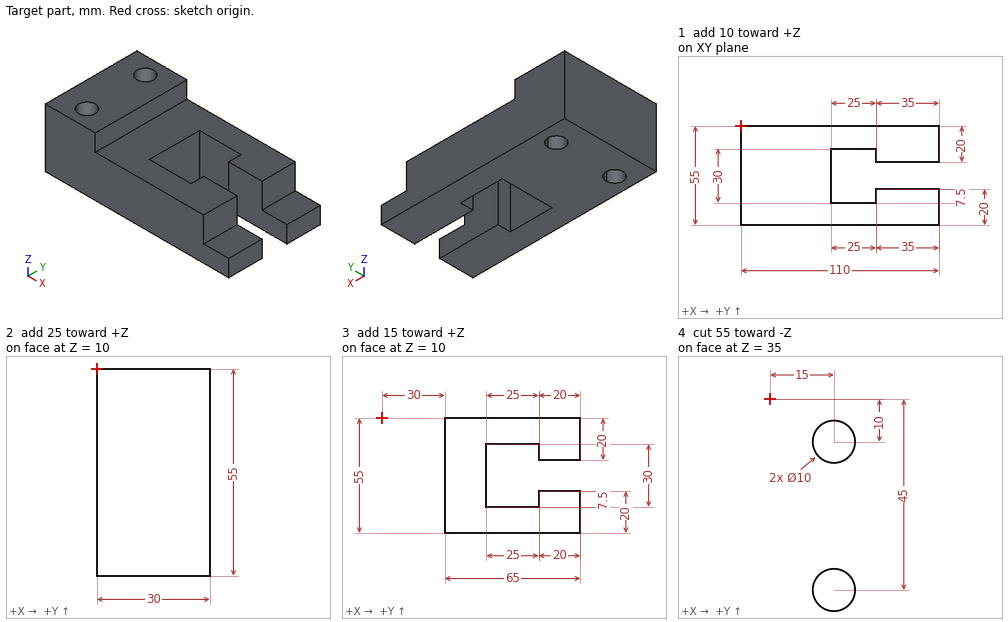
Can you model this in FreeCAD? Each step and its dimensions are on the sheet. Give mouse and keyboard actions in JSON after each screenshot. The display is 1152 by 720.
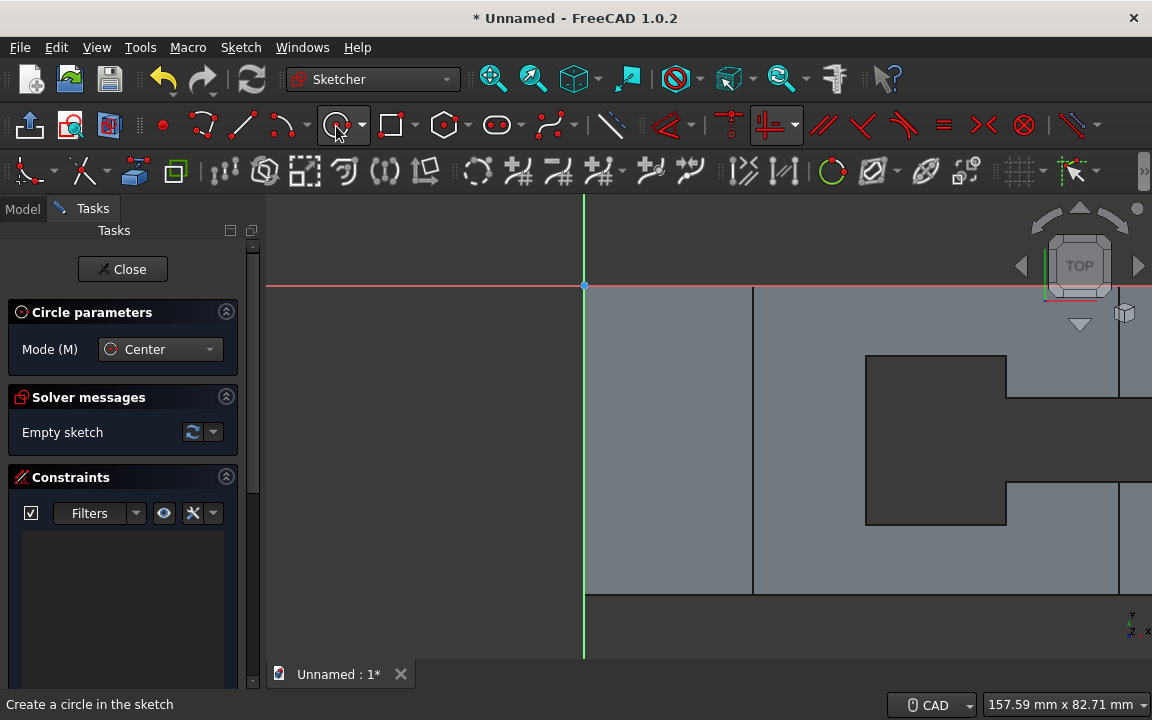
{"action": "left_click", "coordinate": [669, 342]}
{"action": "mouse_move", "coordinate": [689, 322]}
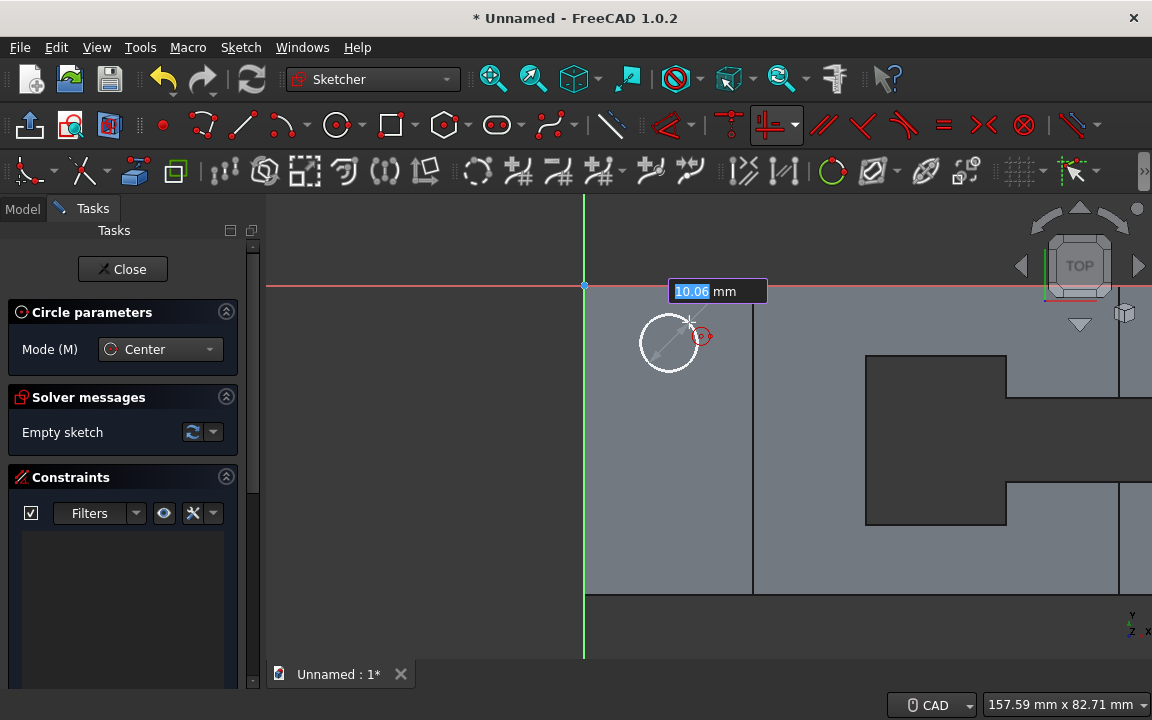
{"action": "type", "text": "10"}
{"action": "key", "text": "Return"}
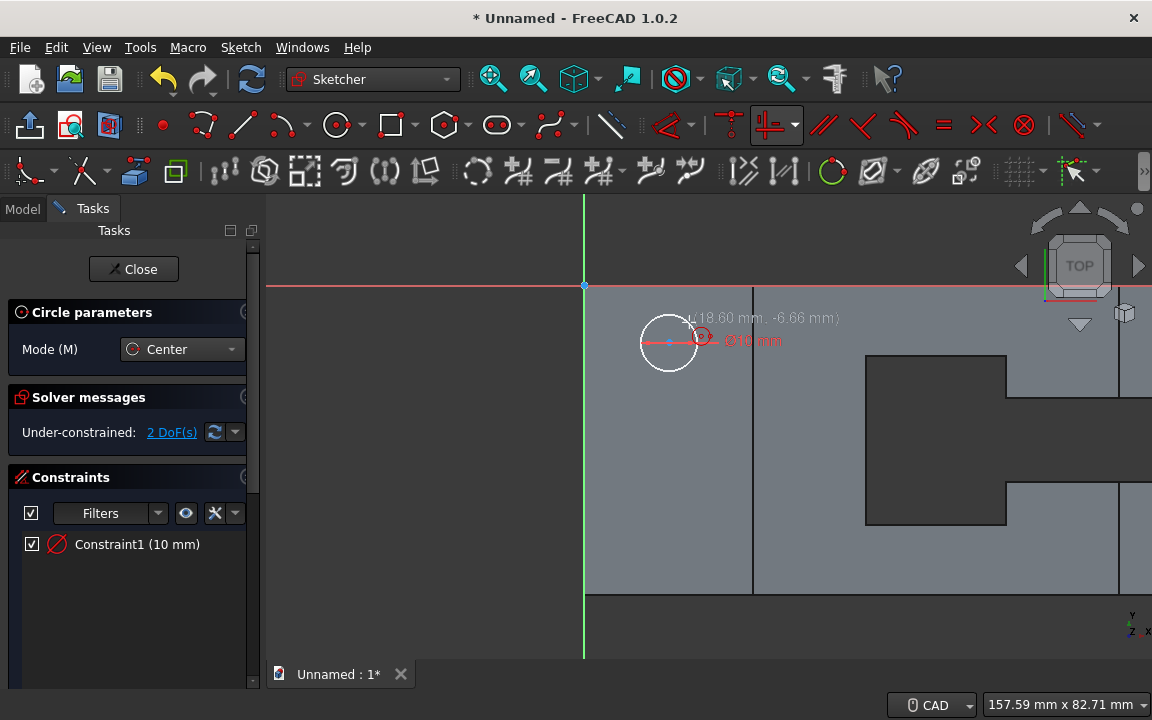
{"action": "left_click", "coordinate": [669, 539]}
{"action": "mouse_move", "coordinate": [689, 519]}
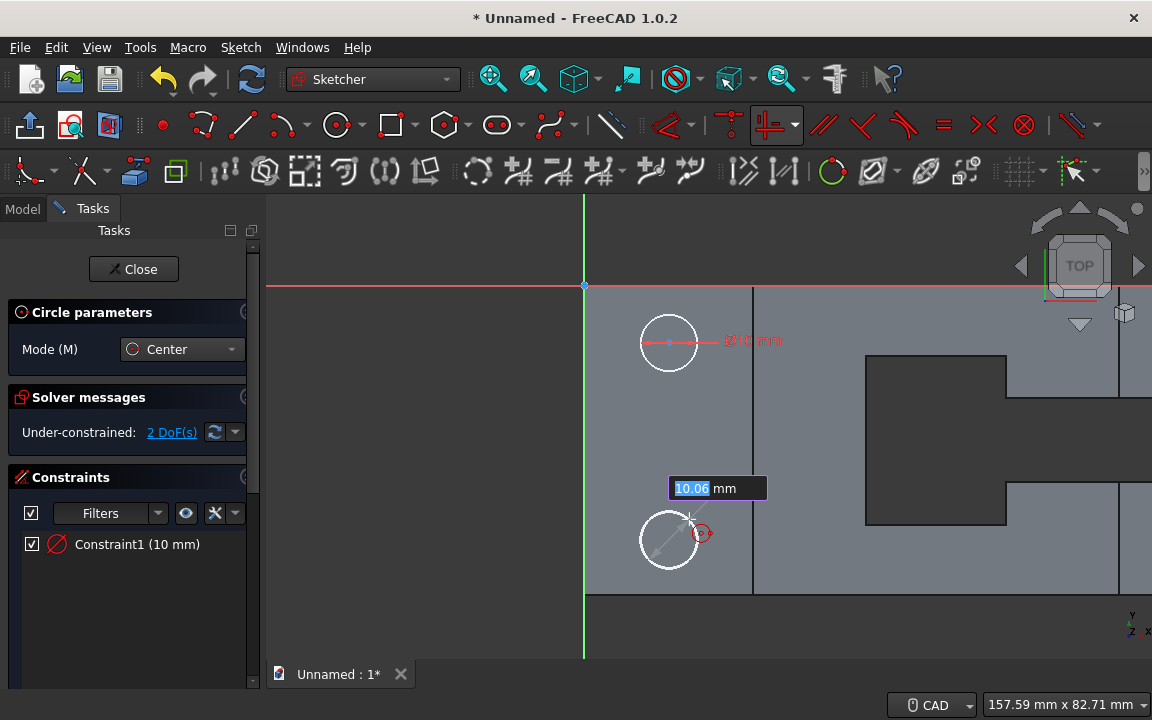
{"action": "type", "text": "10"}
{"action": "key", "text": "Return"}
{"action": "key", "text": "Escape"}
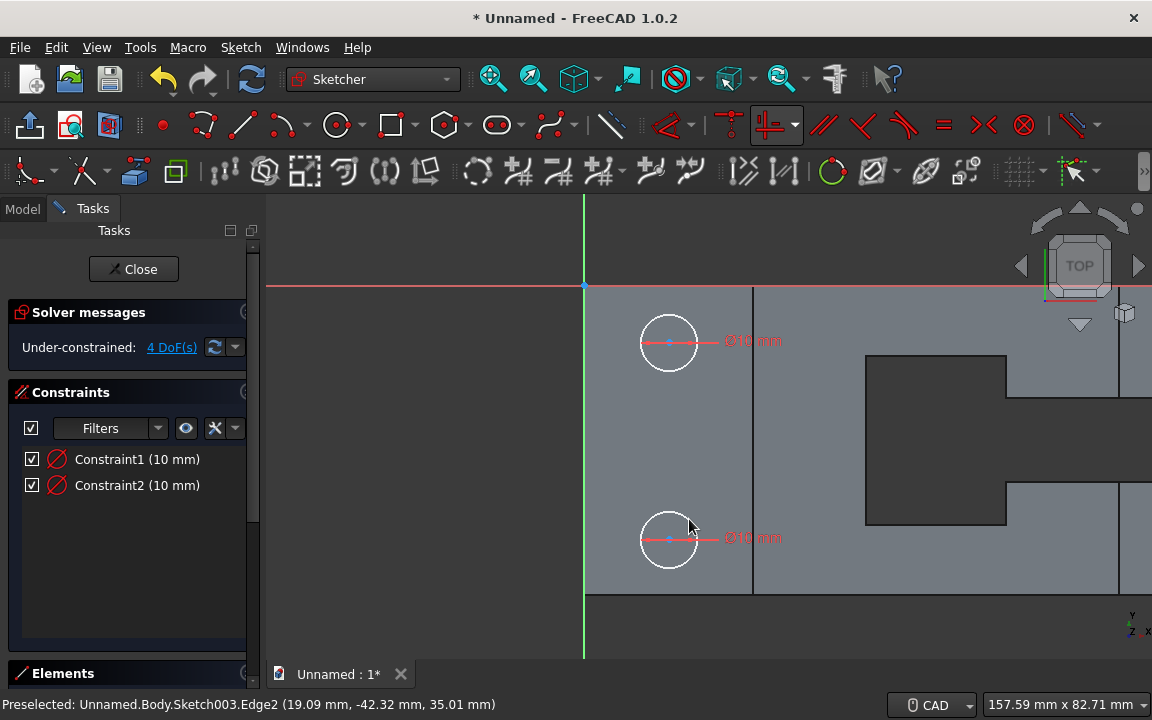
{"action": "left_click", "coordinate": [669, 343]}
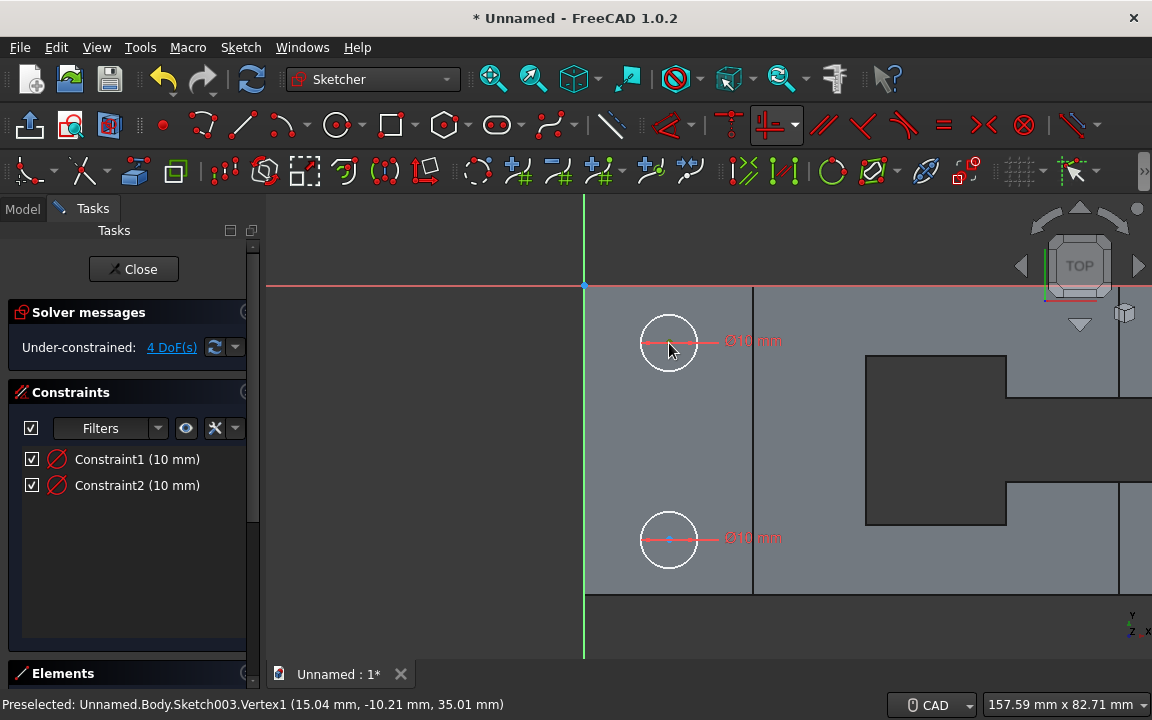
{"action": "left_click", "coordinate": [669, 540]}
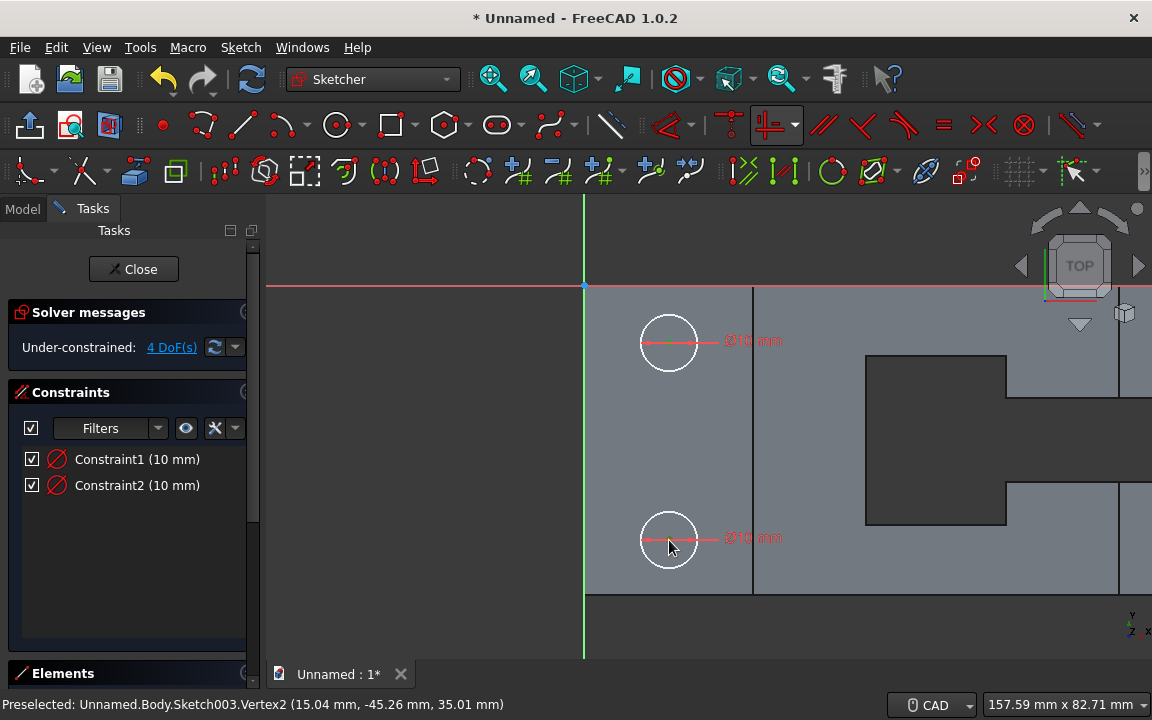
{"action": "left_click", "coordinate": [798, 126]}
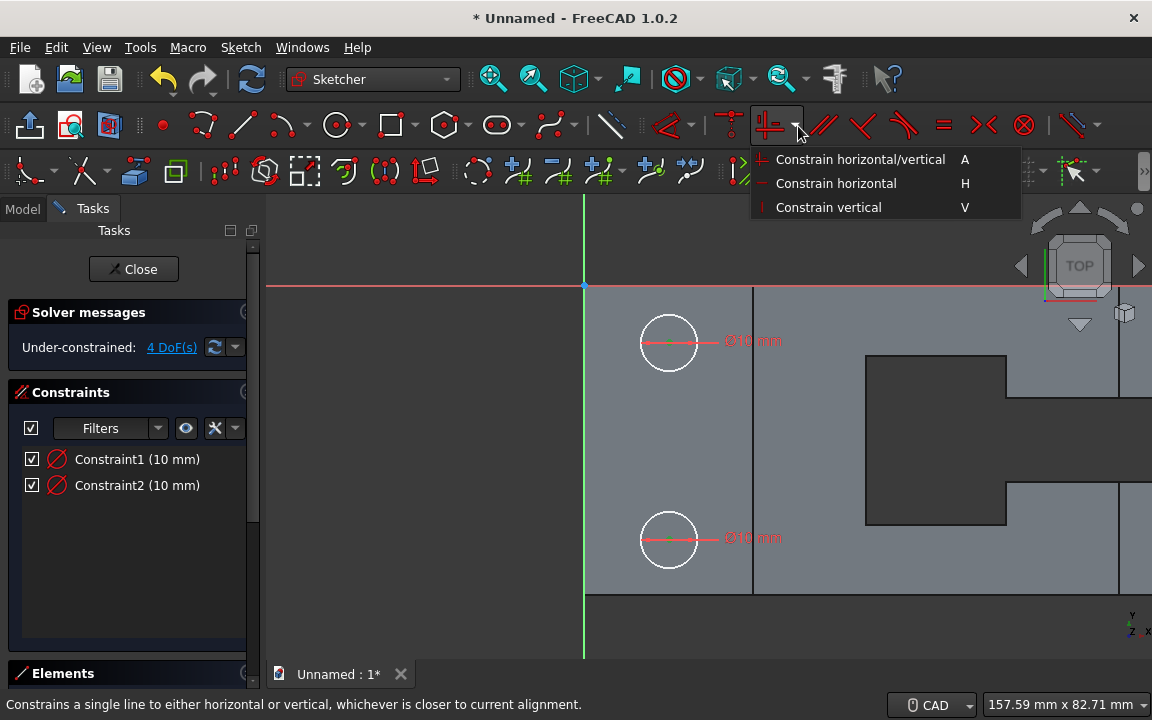
{"action": "left_click", "coordinate": [886, 207]}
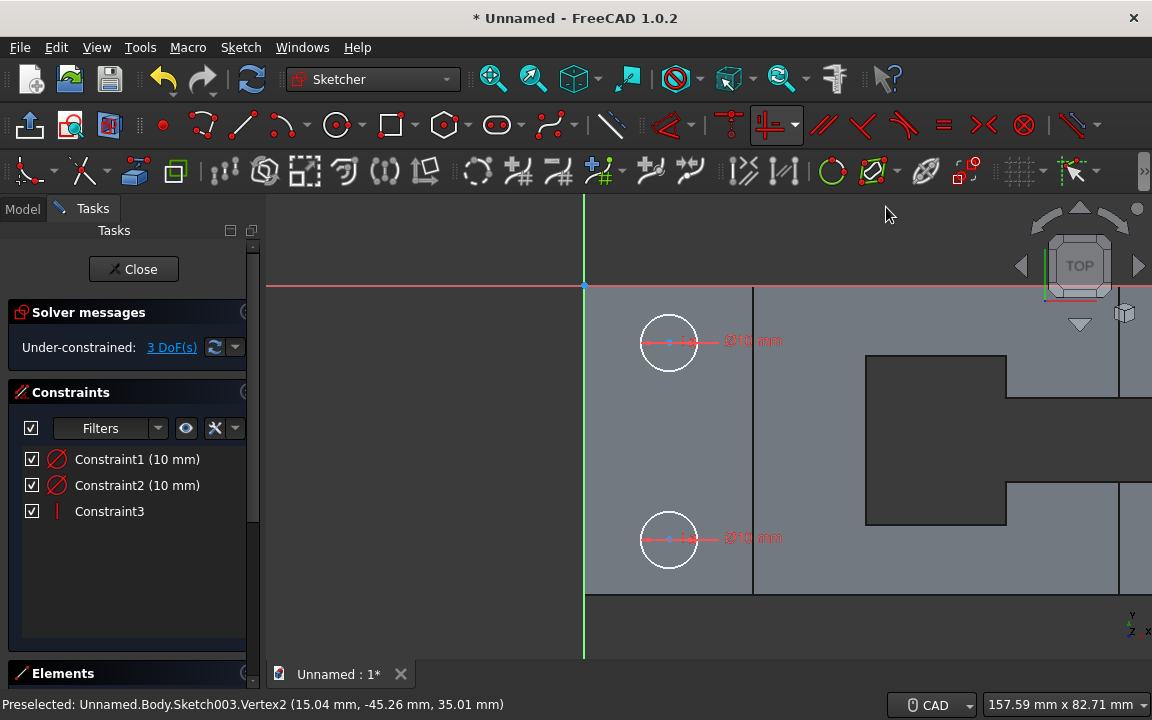
{"action": "left_click", "coordinate": [666, 126]}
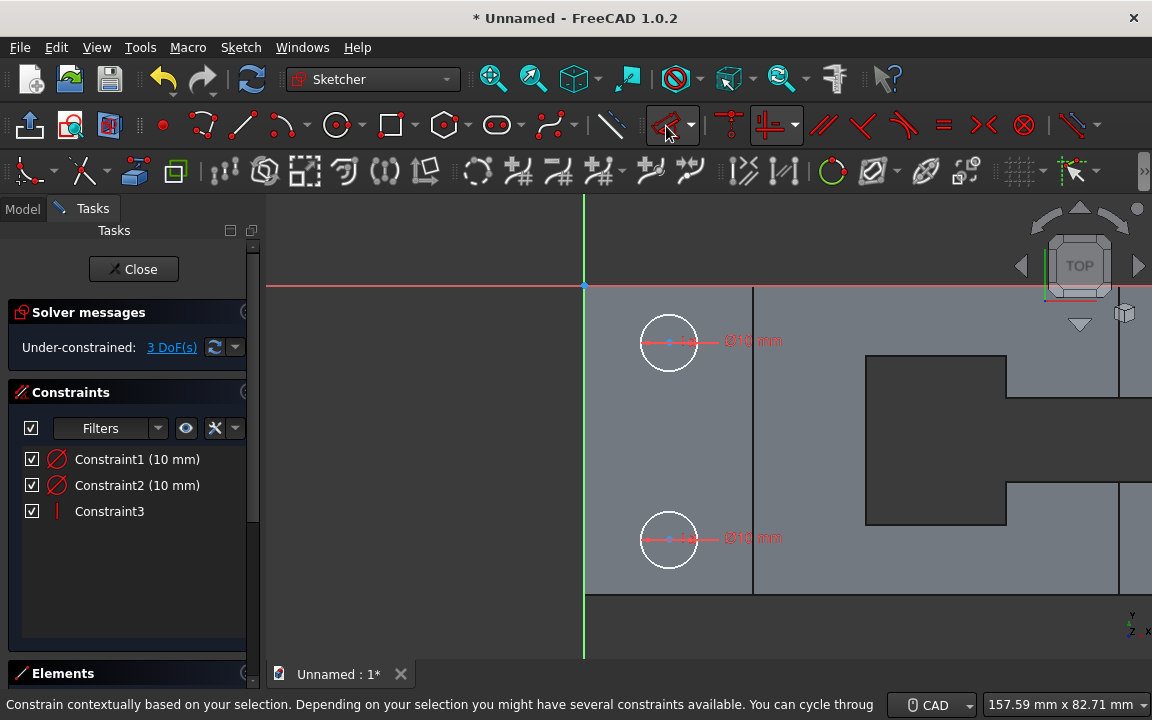
{"action": "left_click", "coordinate": [669, 343]}
{"action": "left_click", "coordinate": [627, 252]}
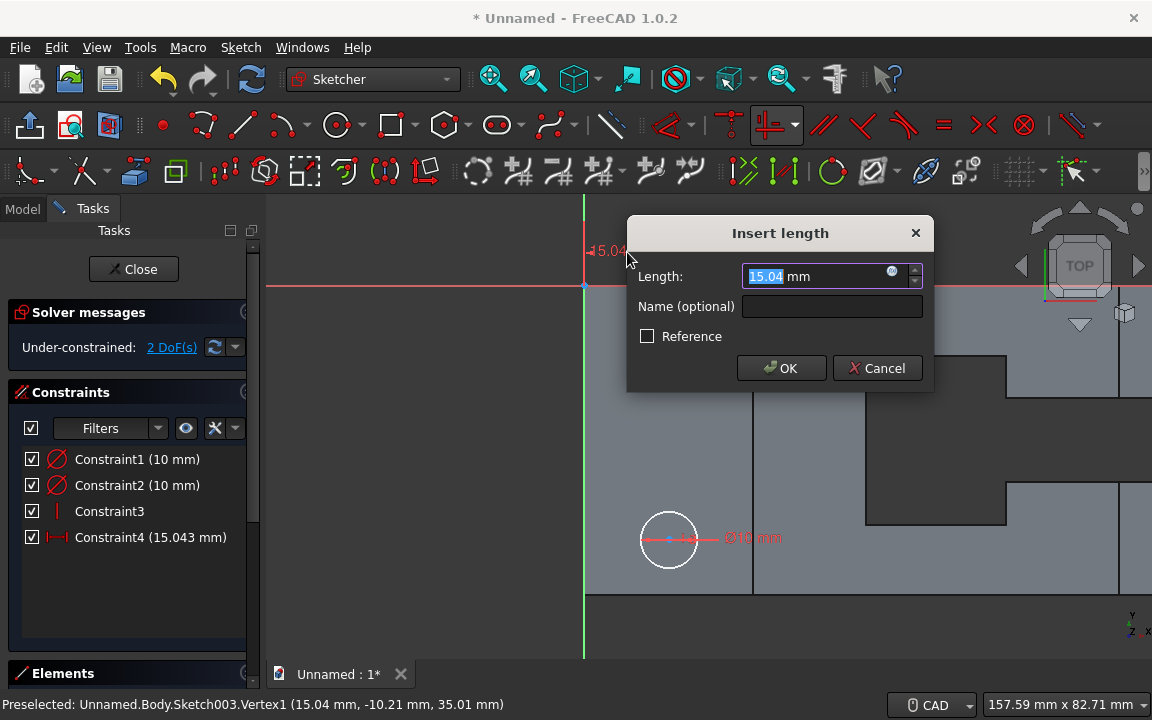
{"action": "type", "text": "15"}
{"action": "key", "text": "Return"}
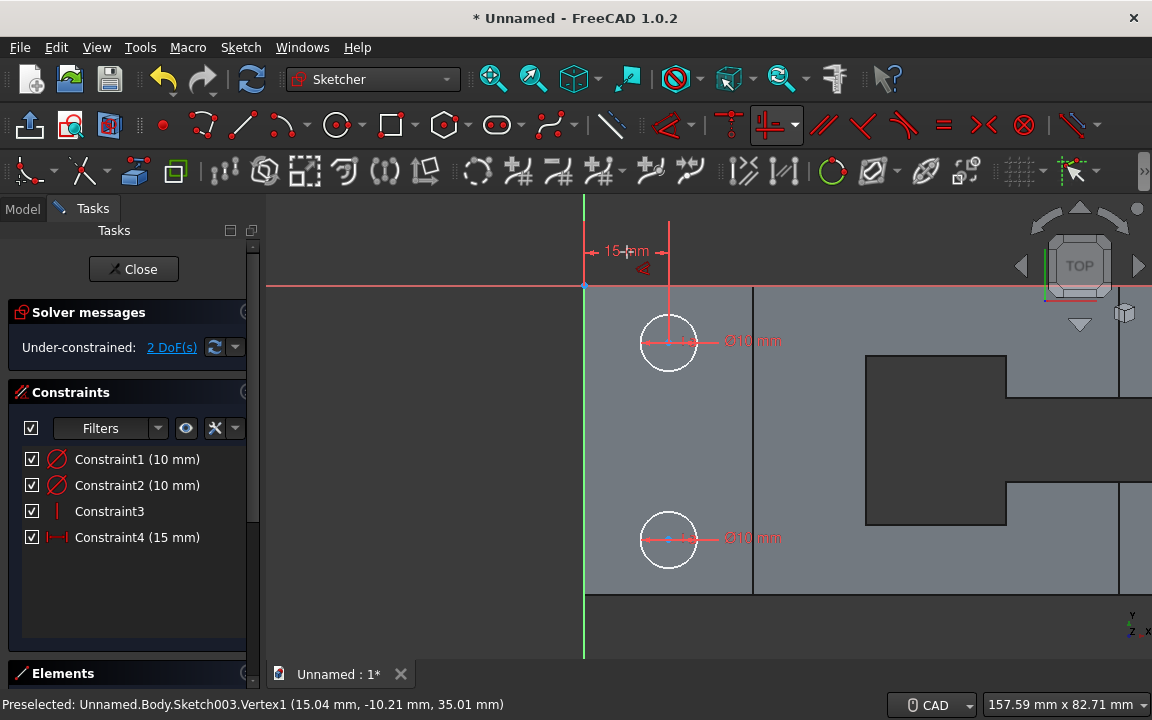
{"action": "left_click", "coordinate": [669, 343]}
{"action": "left_click", "coordinate": [550, 314]}